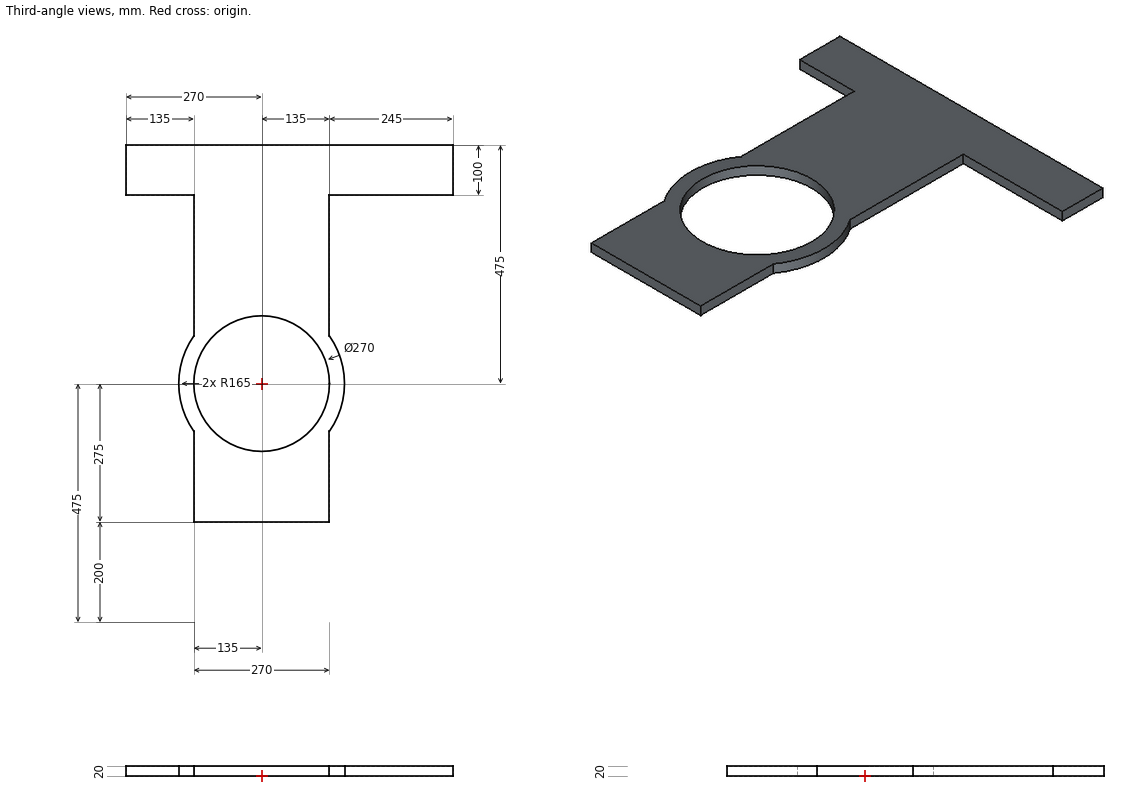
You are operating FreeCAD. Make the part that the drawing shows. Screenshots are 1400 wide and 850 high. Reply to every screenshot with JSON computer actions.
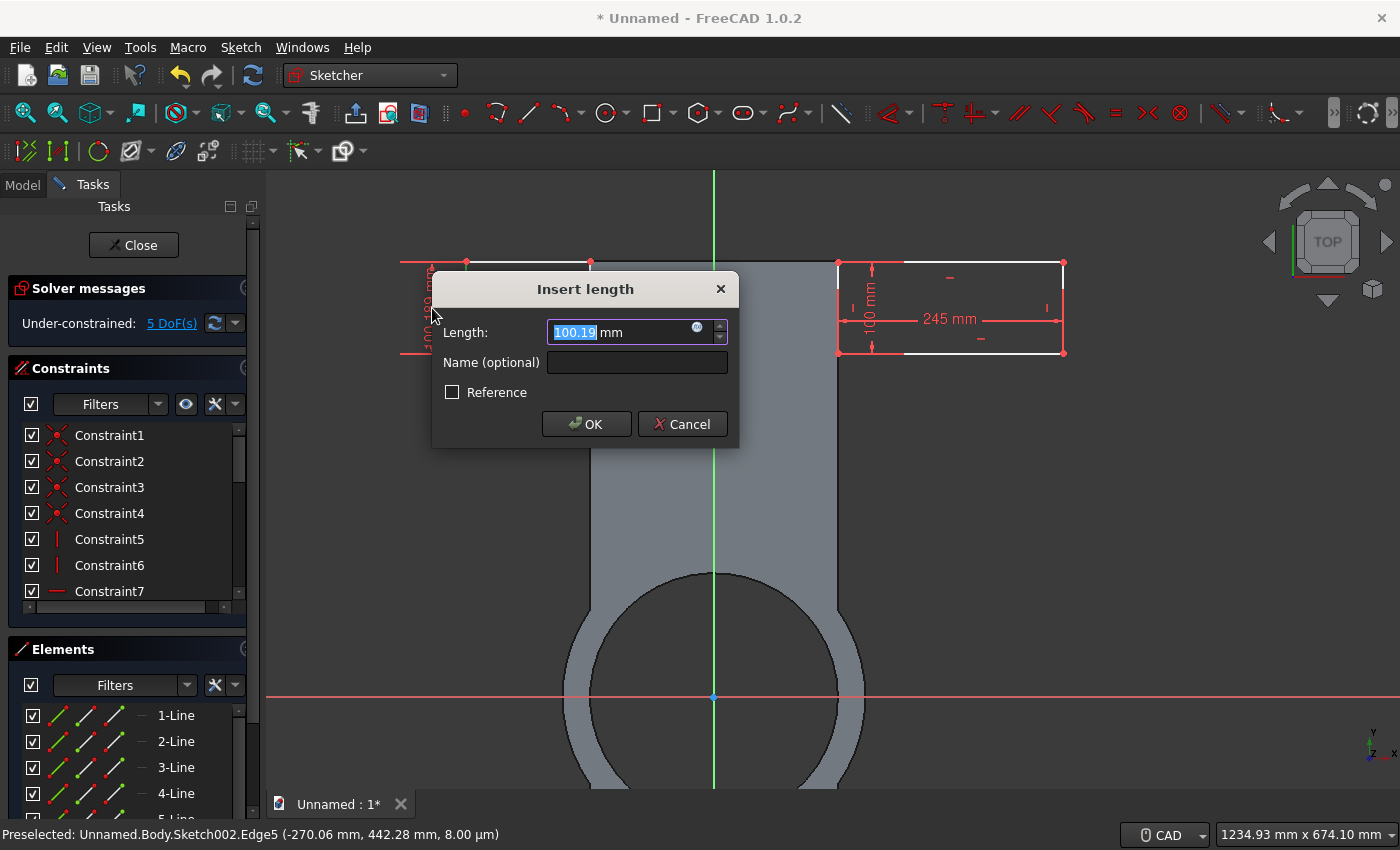
{"action": "type", "text": "100"}
{"action": "key", "text": "Return"}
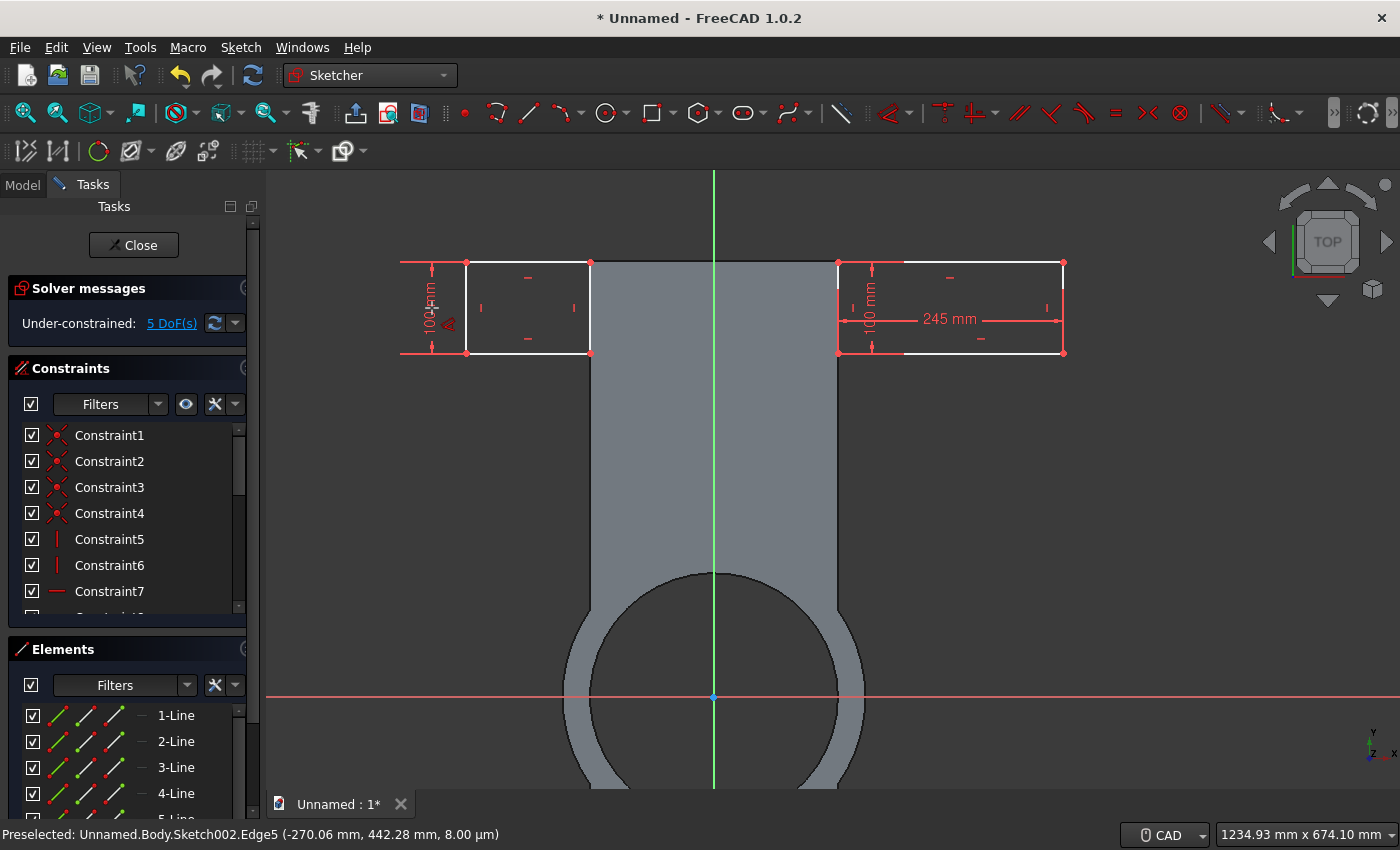
{"action": "left_click", "coordinate": [503, 354]}
{"action": "left_click", "coordinate": [528, 320]}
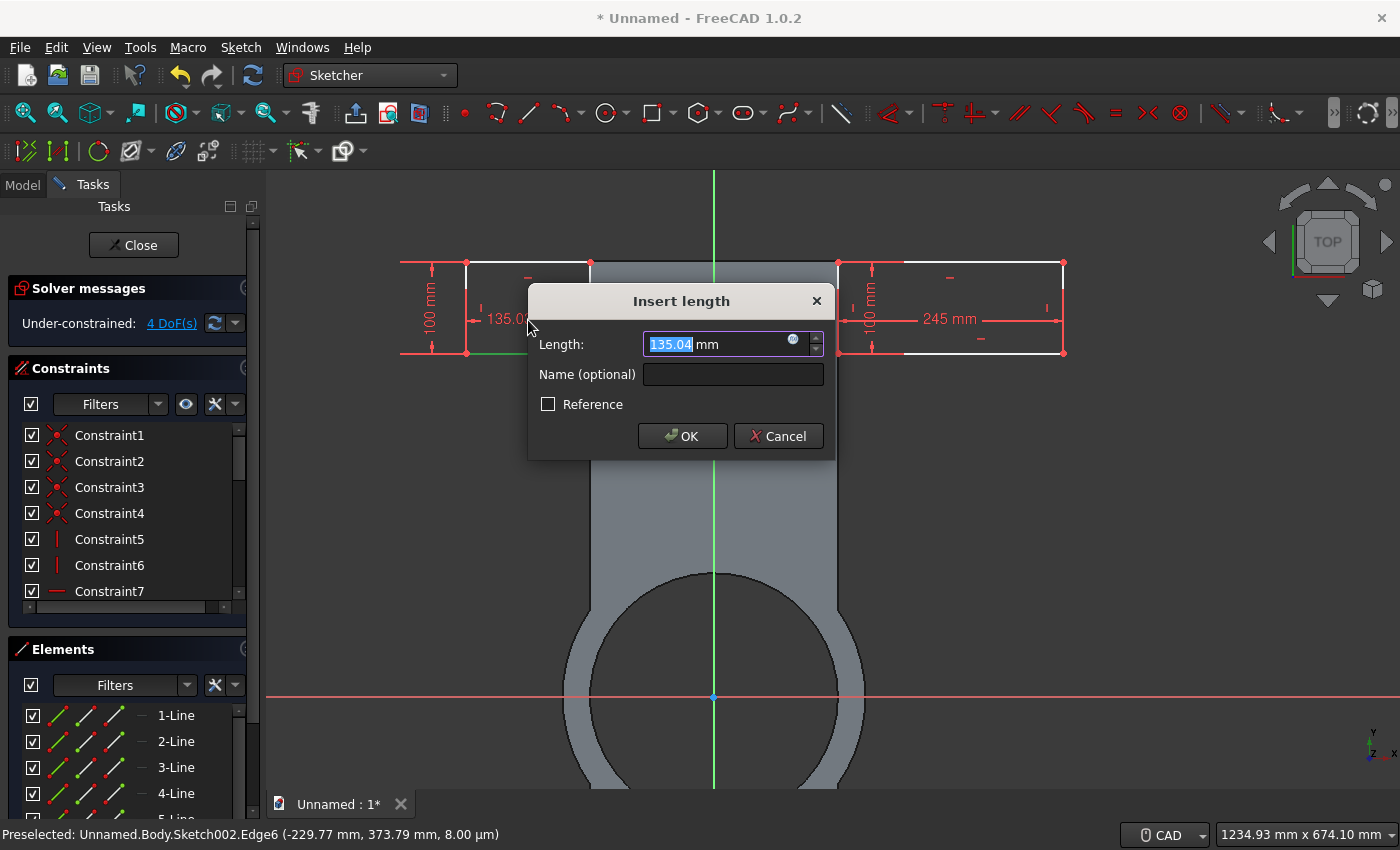
{"action": "type", "text": "135"}
{"action": "key", "text": "Return"}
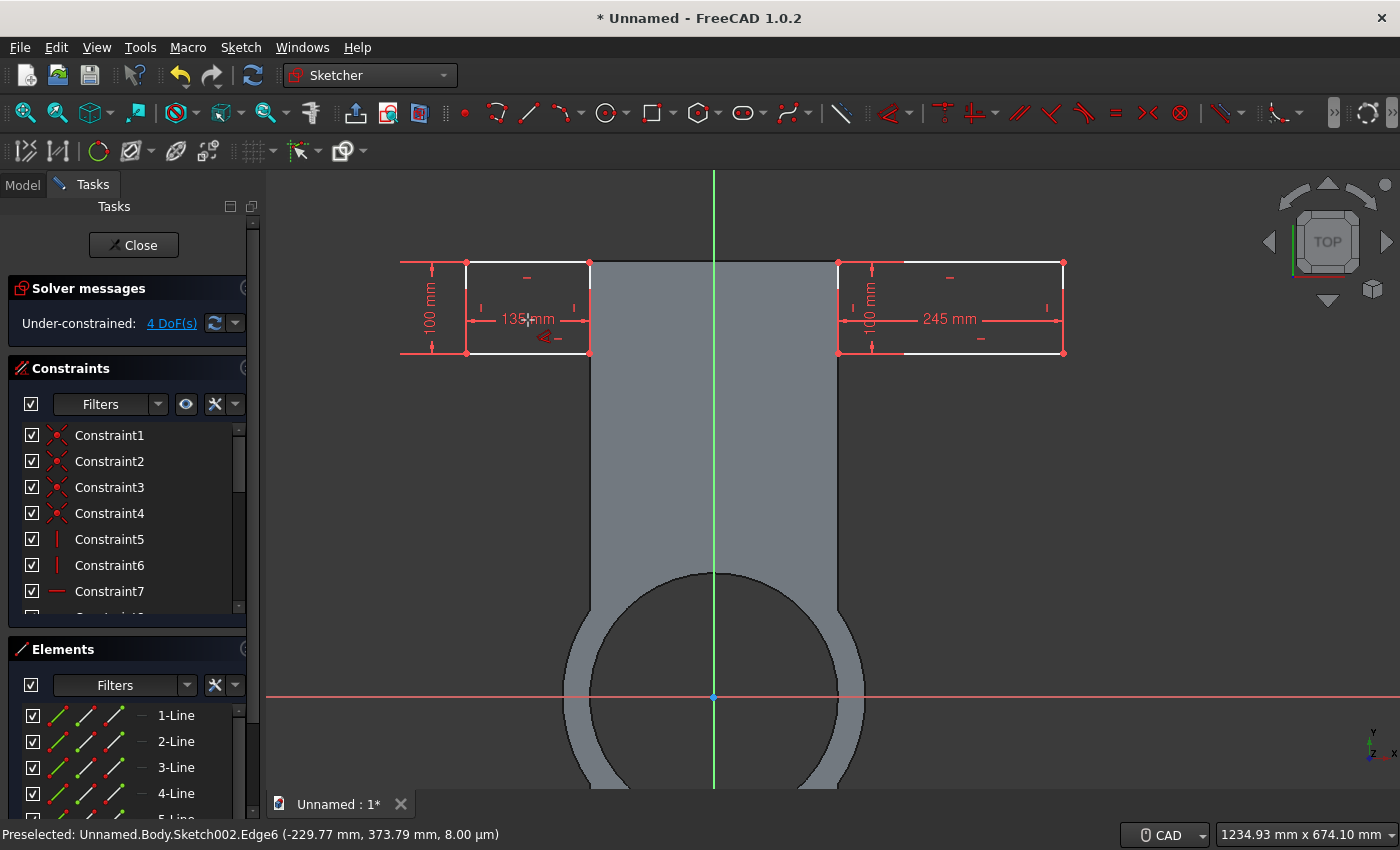
{"action": "left_click", "coordinate": [838, 262]}
{"action": "left_click", "coordinate": [776, 731]}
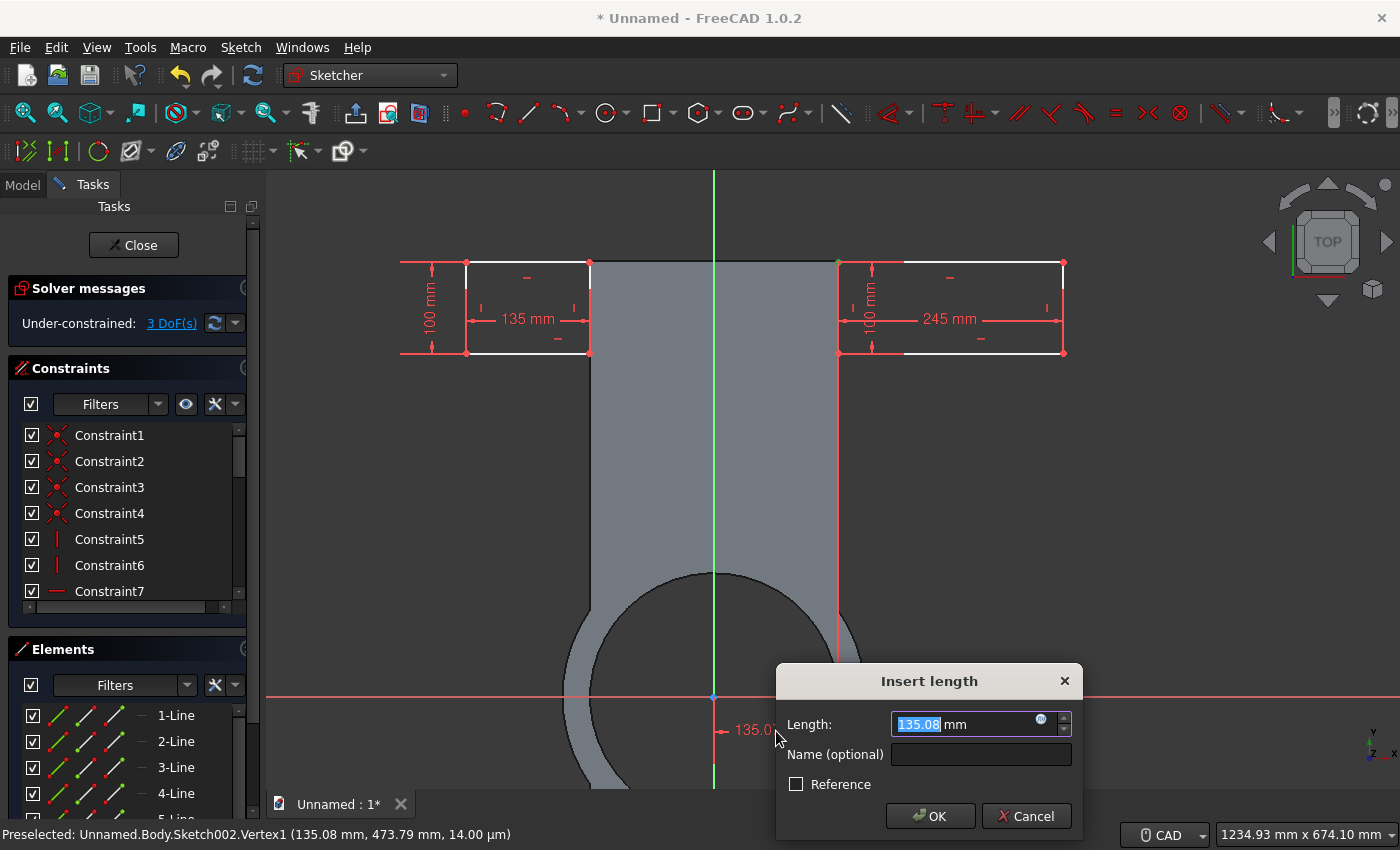
{"action": "type", "text": "135"}
{"action": "key", "text": "Return"}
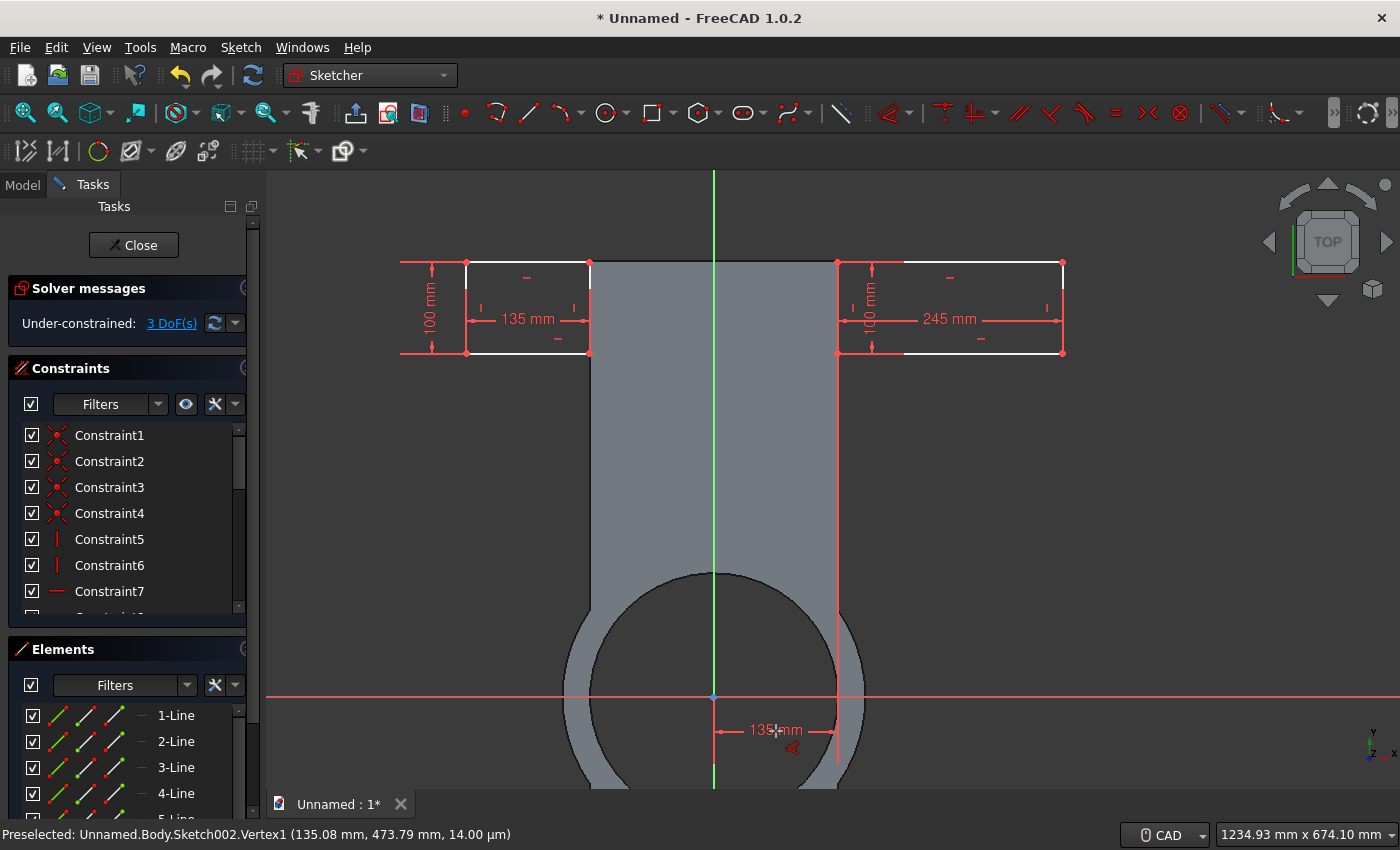
{"action": "left_click", "coordinate": [838, 262]}
{"action": "left_click", "coordinate": [872, 480]}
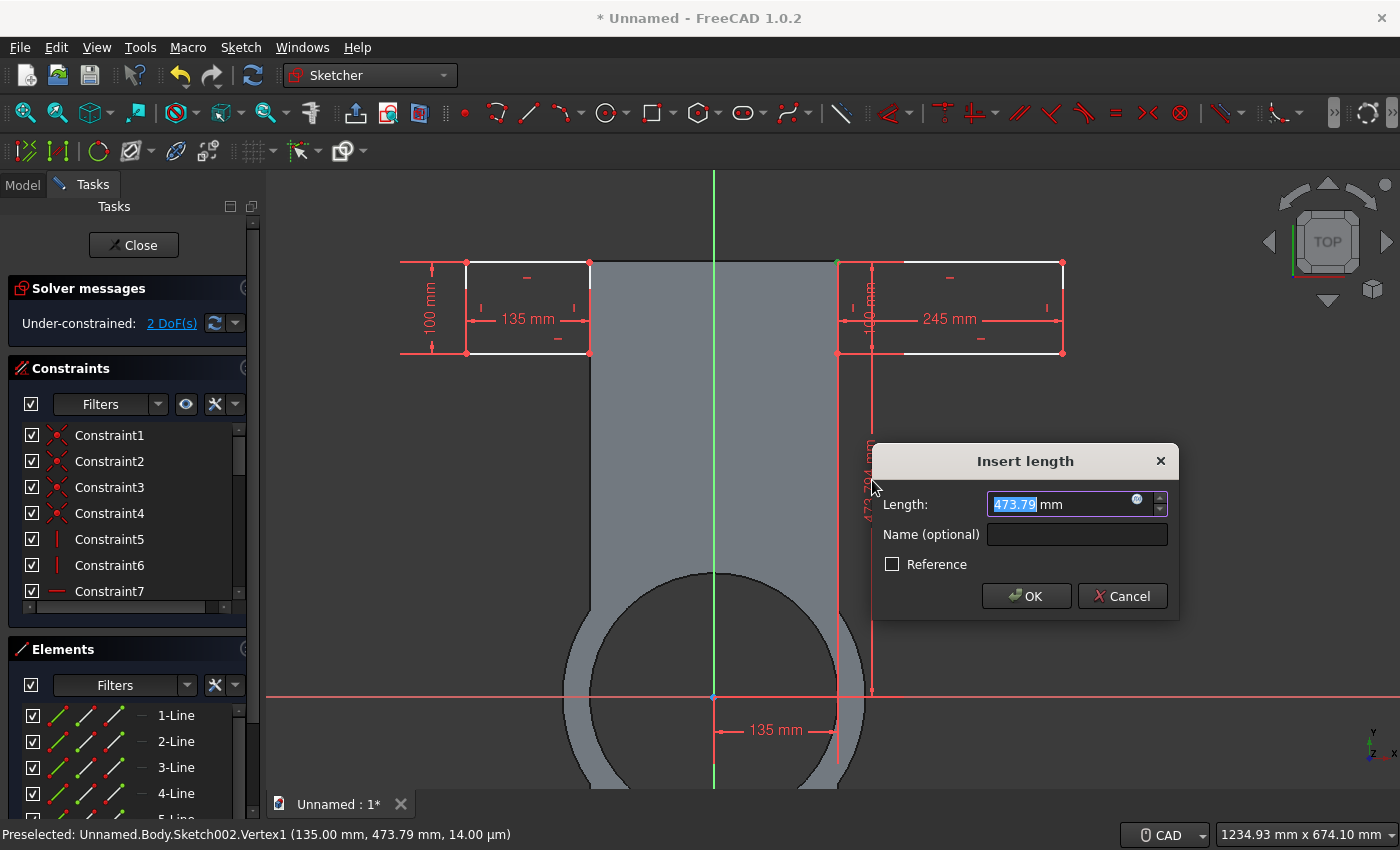
{"action": "type", "text": "475"}
{"action": "key", "text": "Return"}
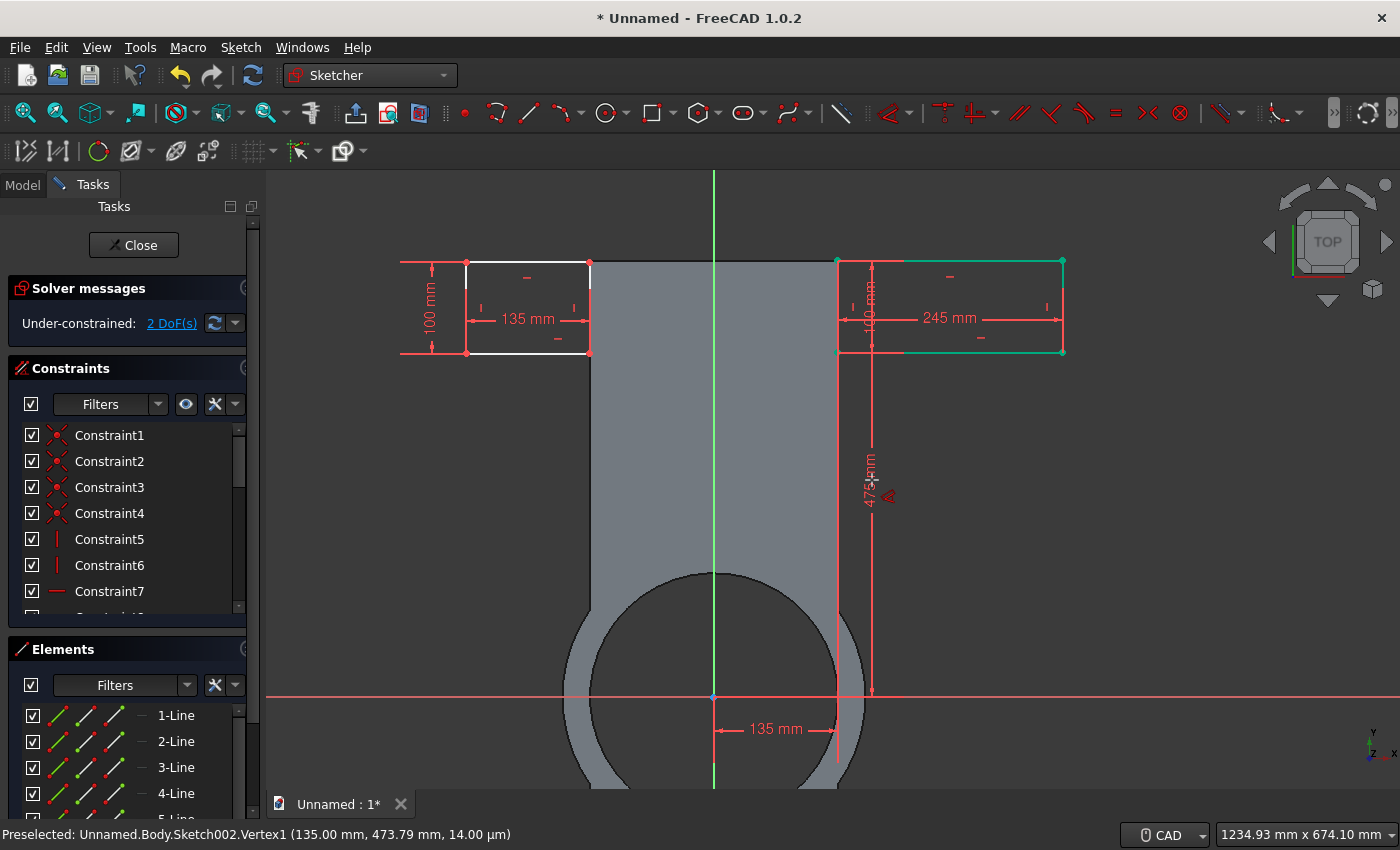
{"action": "left_click", "coordinate": [466, 262]}
{"action": "left_click", "coordinate": [590, 731]}